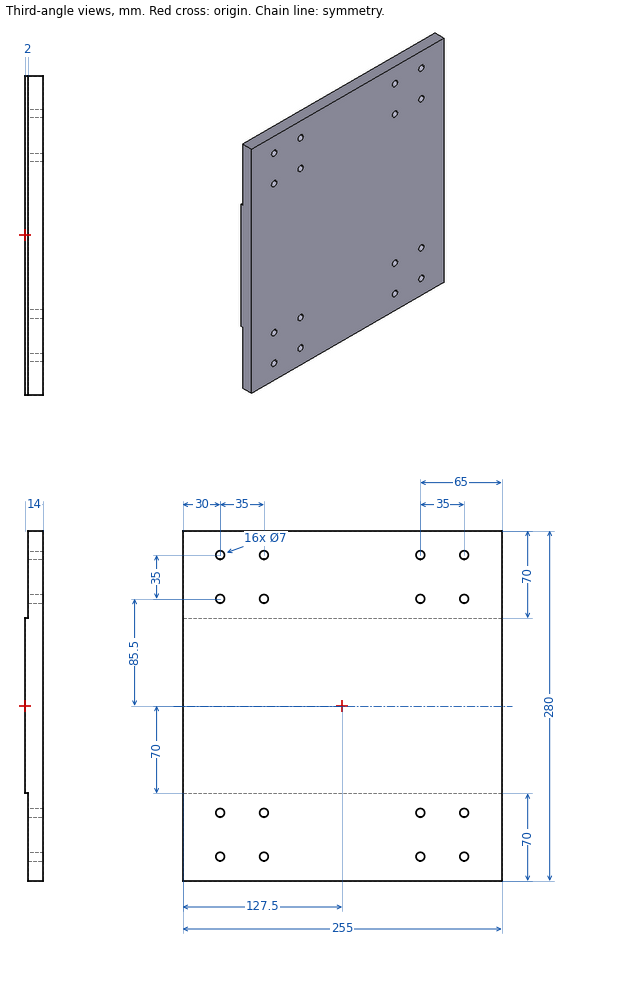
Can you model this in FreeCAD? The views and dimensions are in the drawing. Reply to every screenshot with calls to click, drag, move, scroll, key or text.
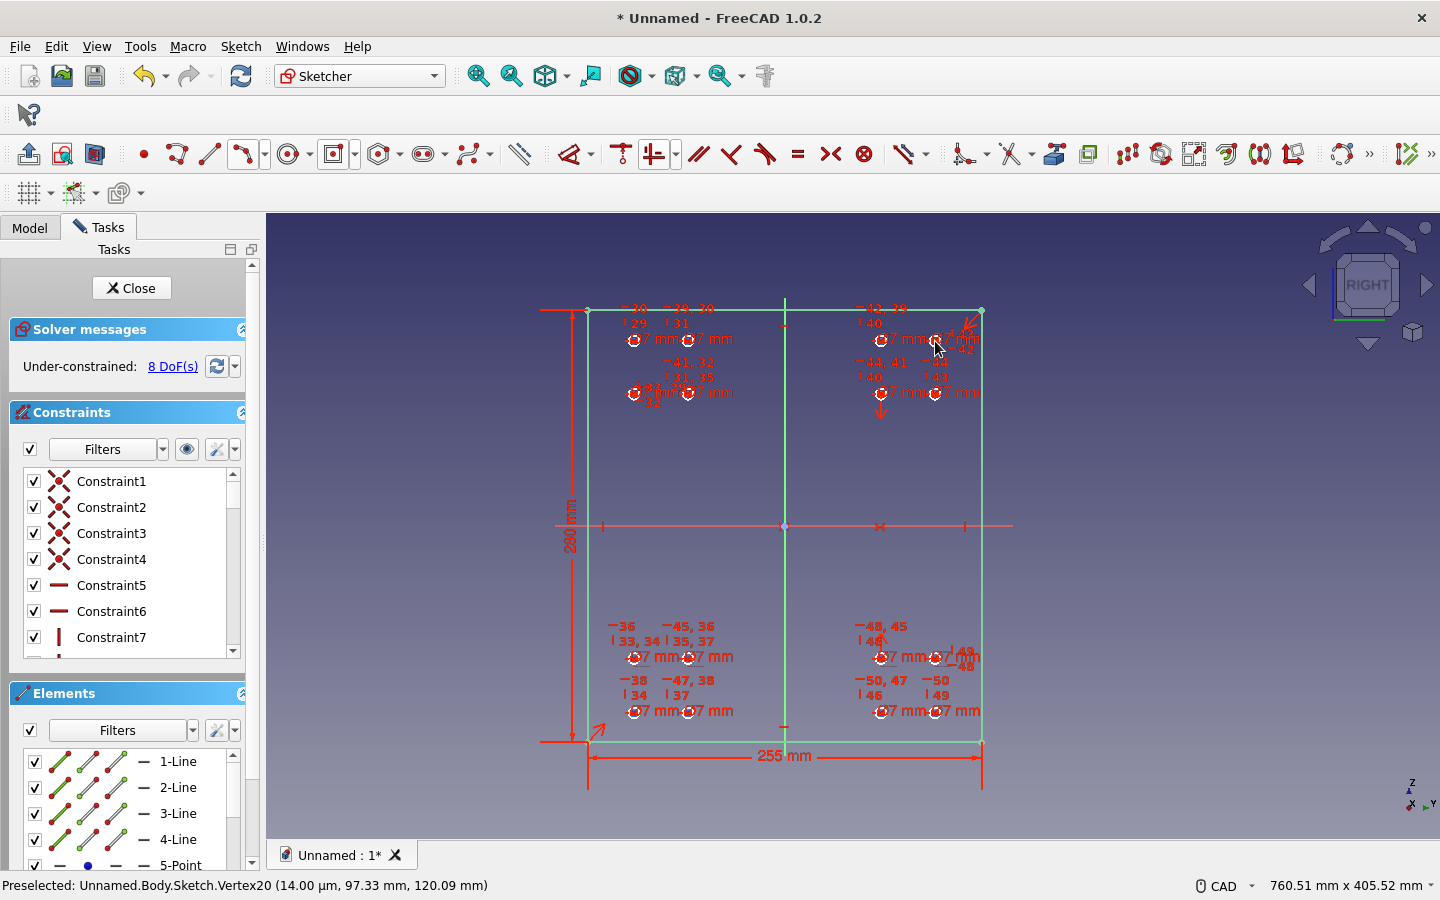
click(935, 713)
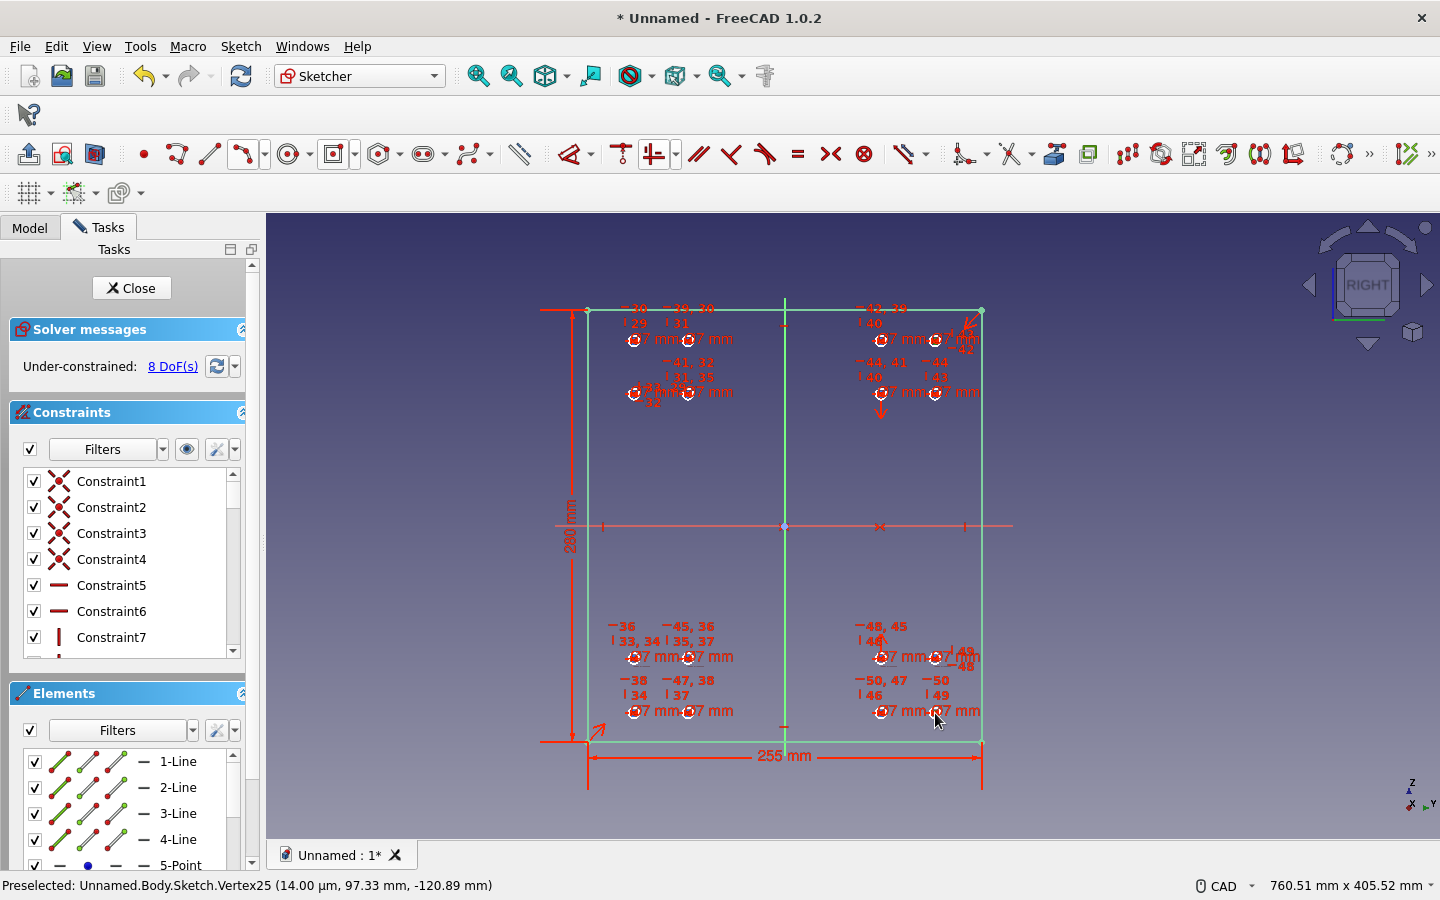
click(644, 526)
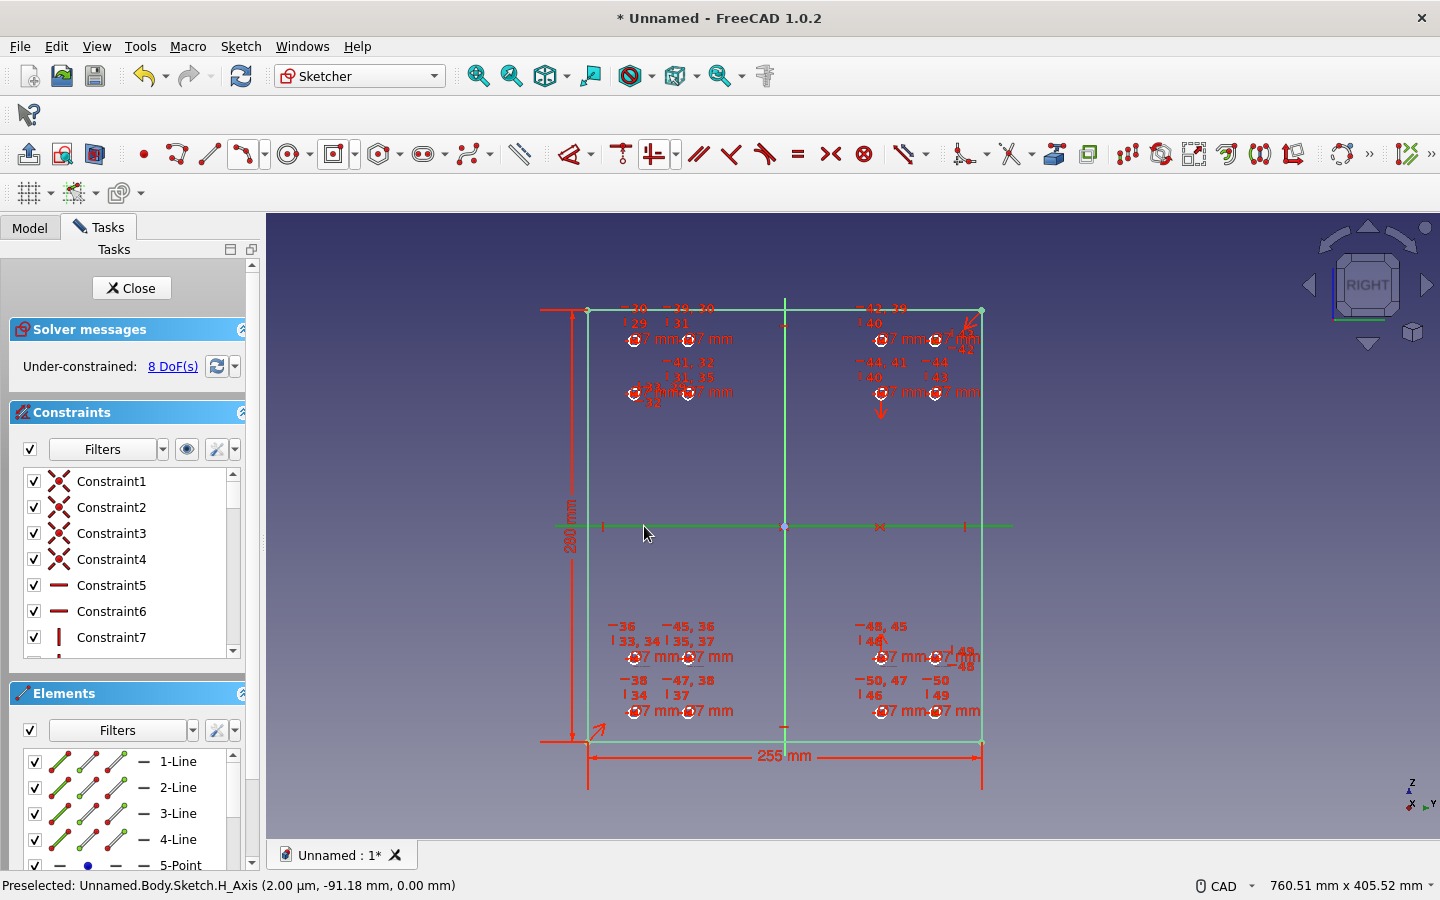
click(831, 154)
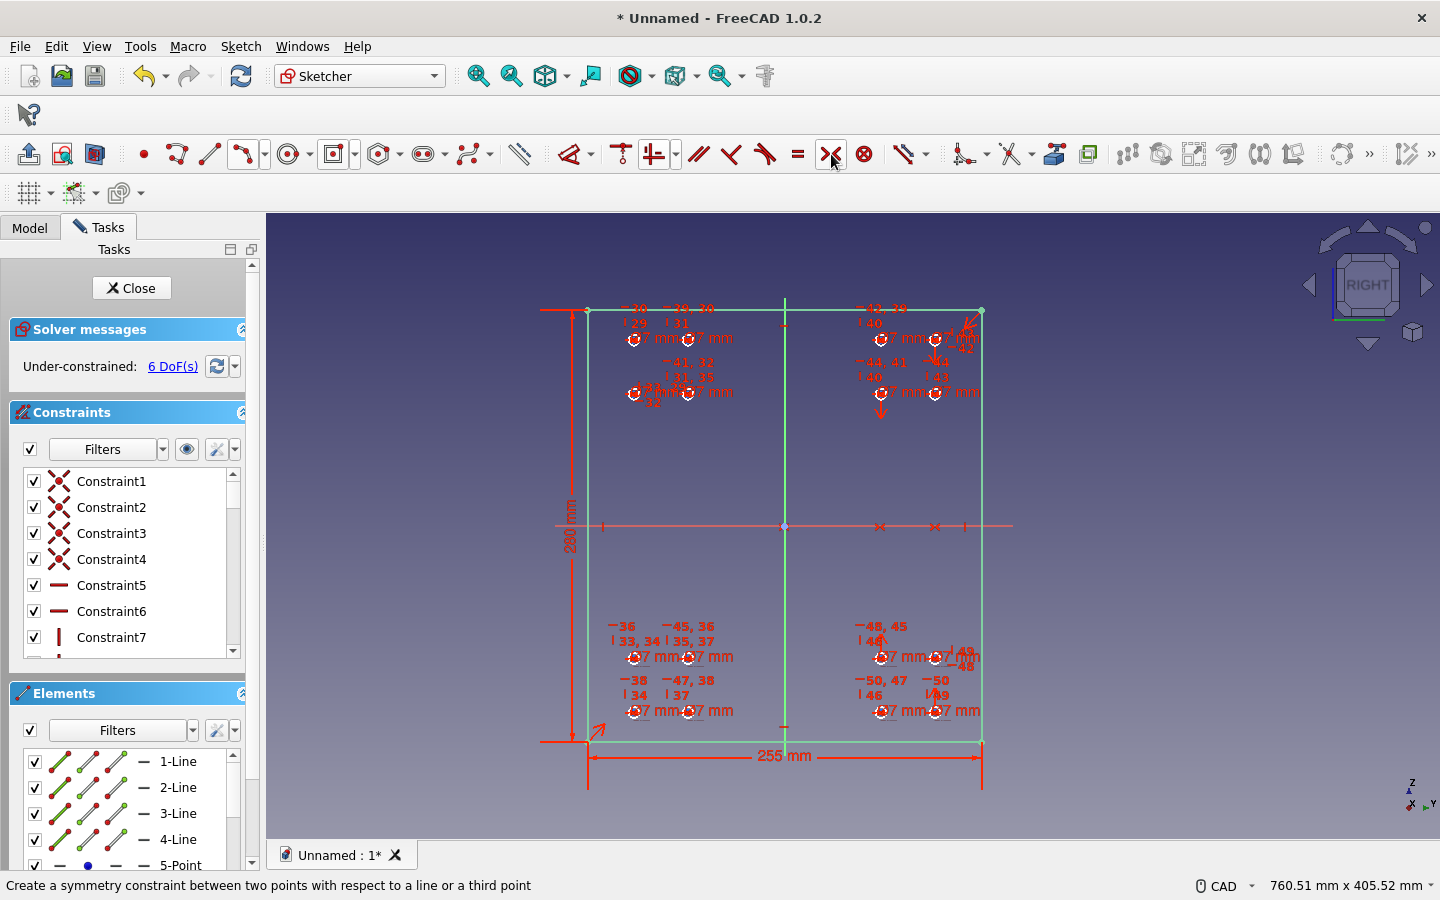
click(588, 310)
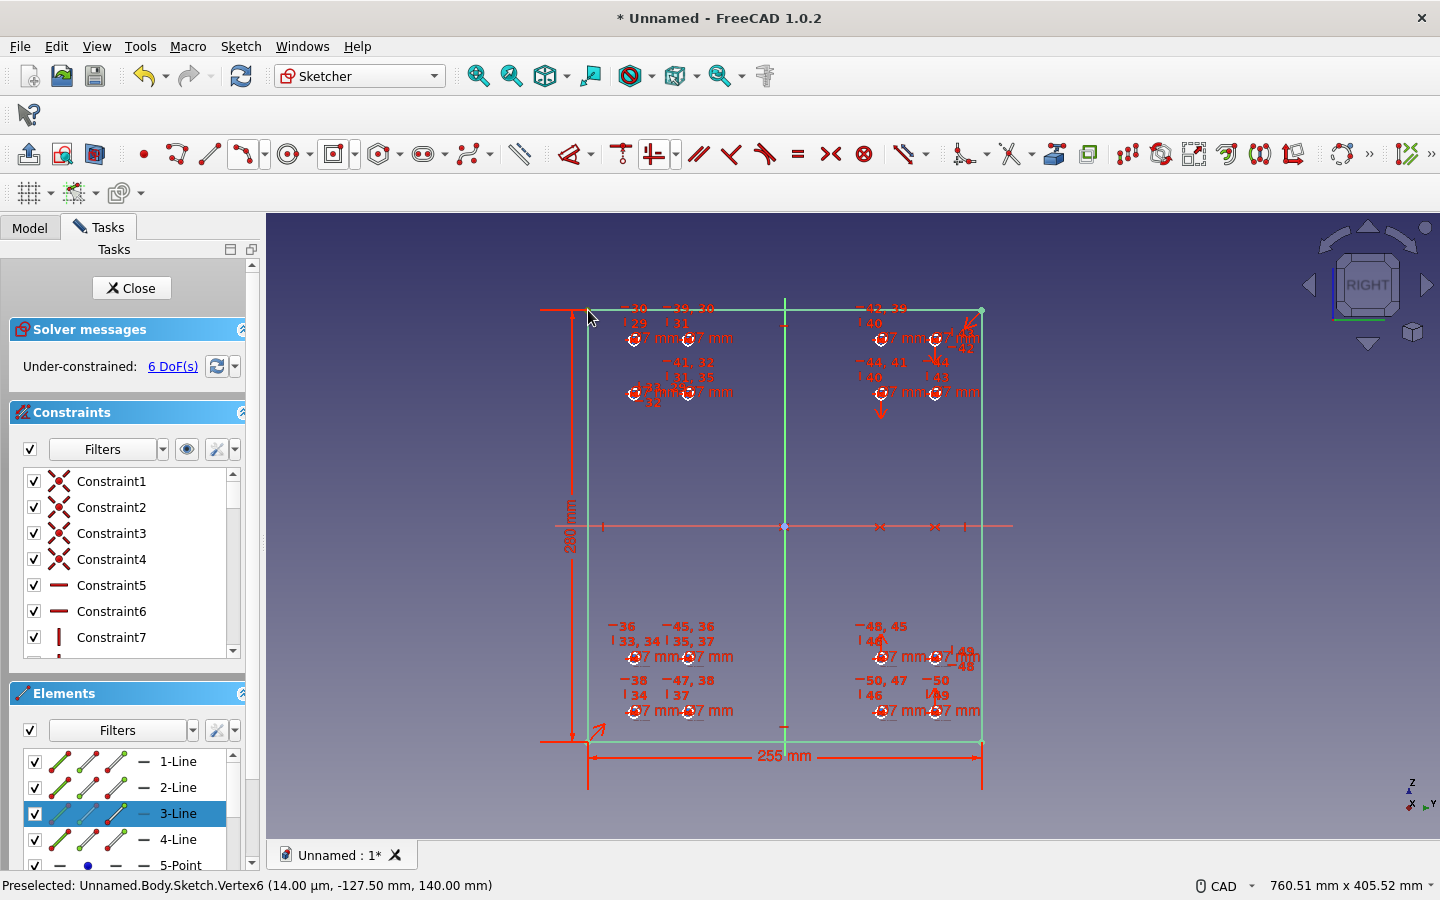
click(634, 340)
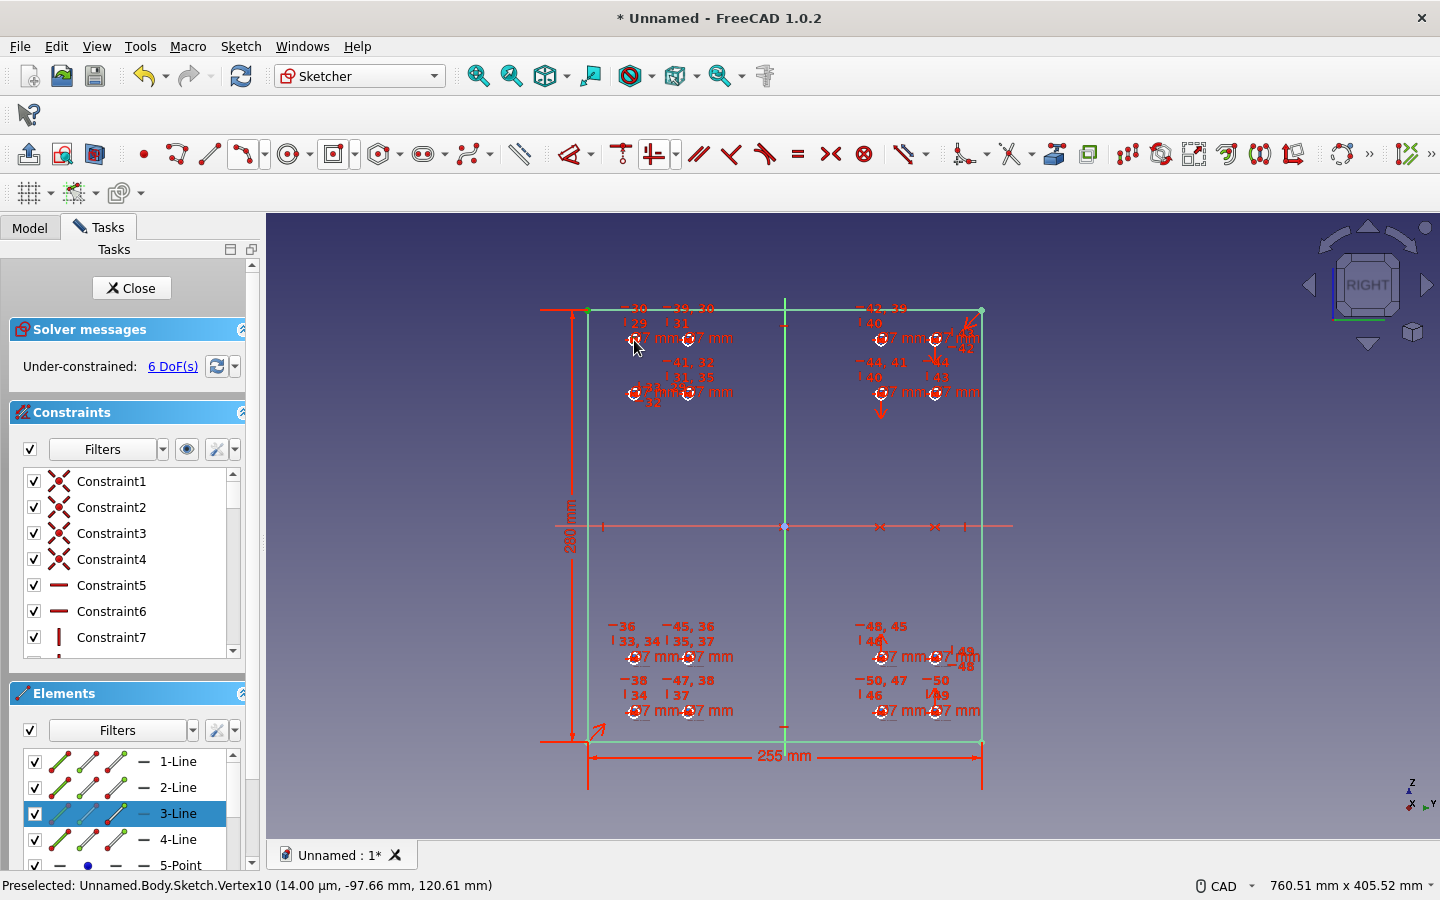
click(590, 154)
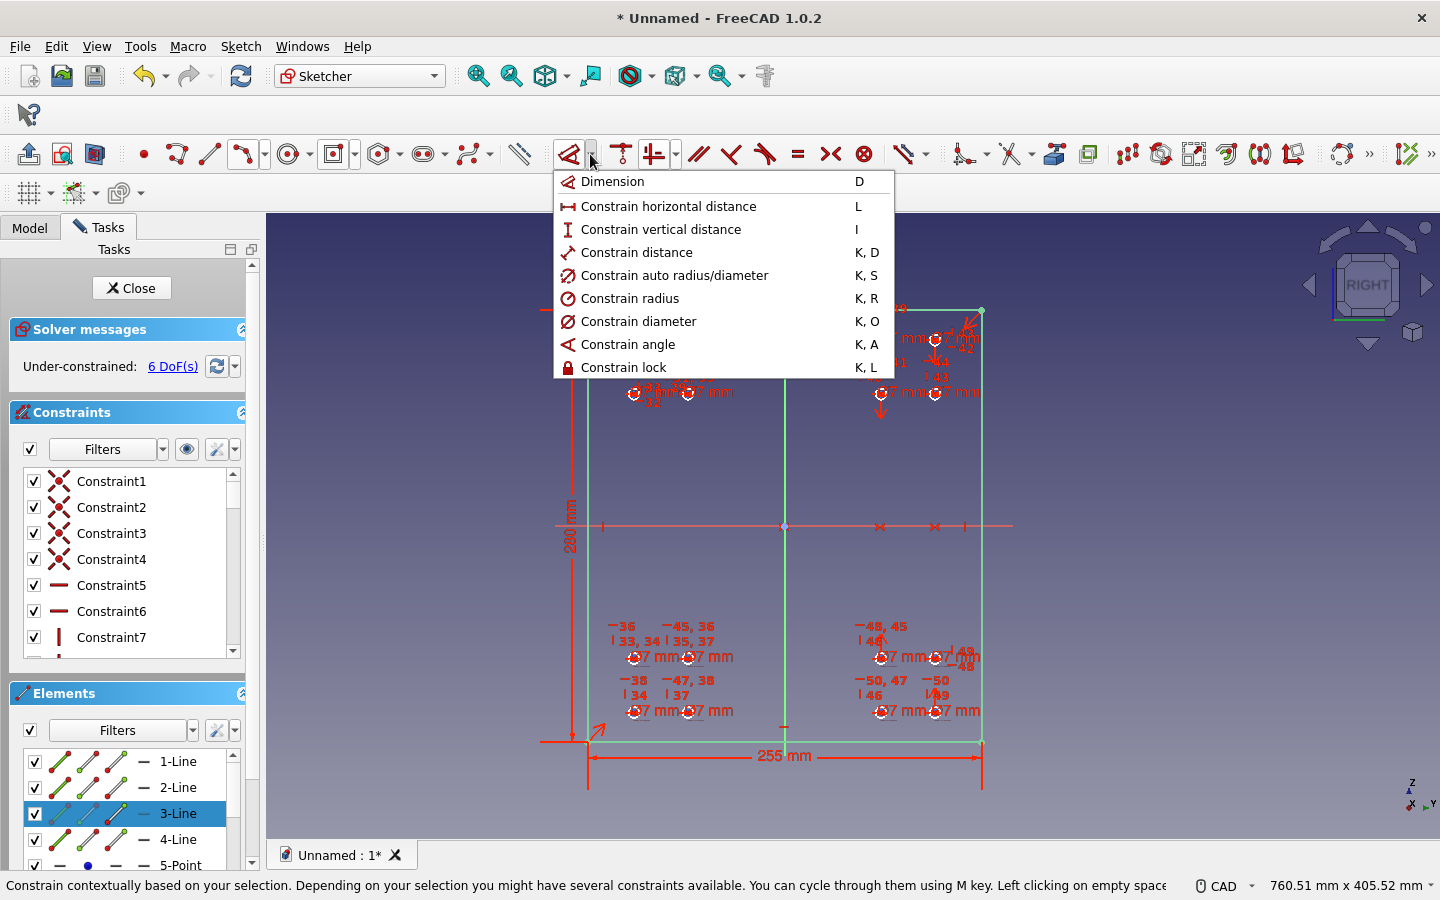
click(724, 206)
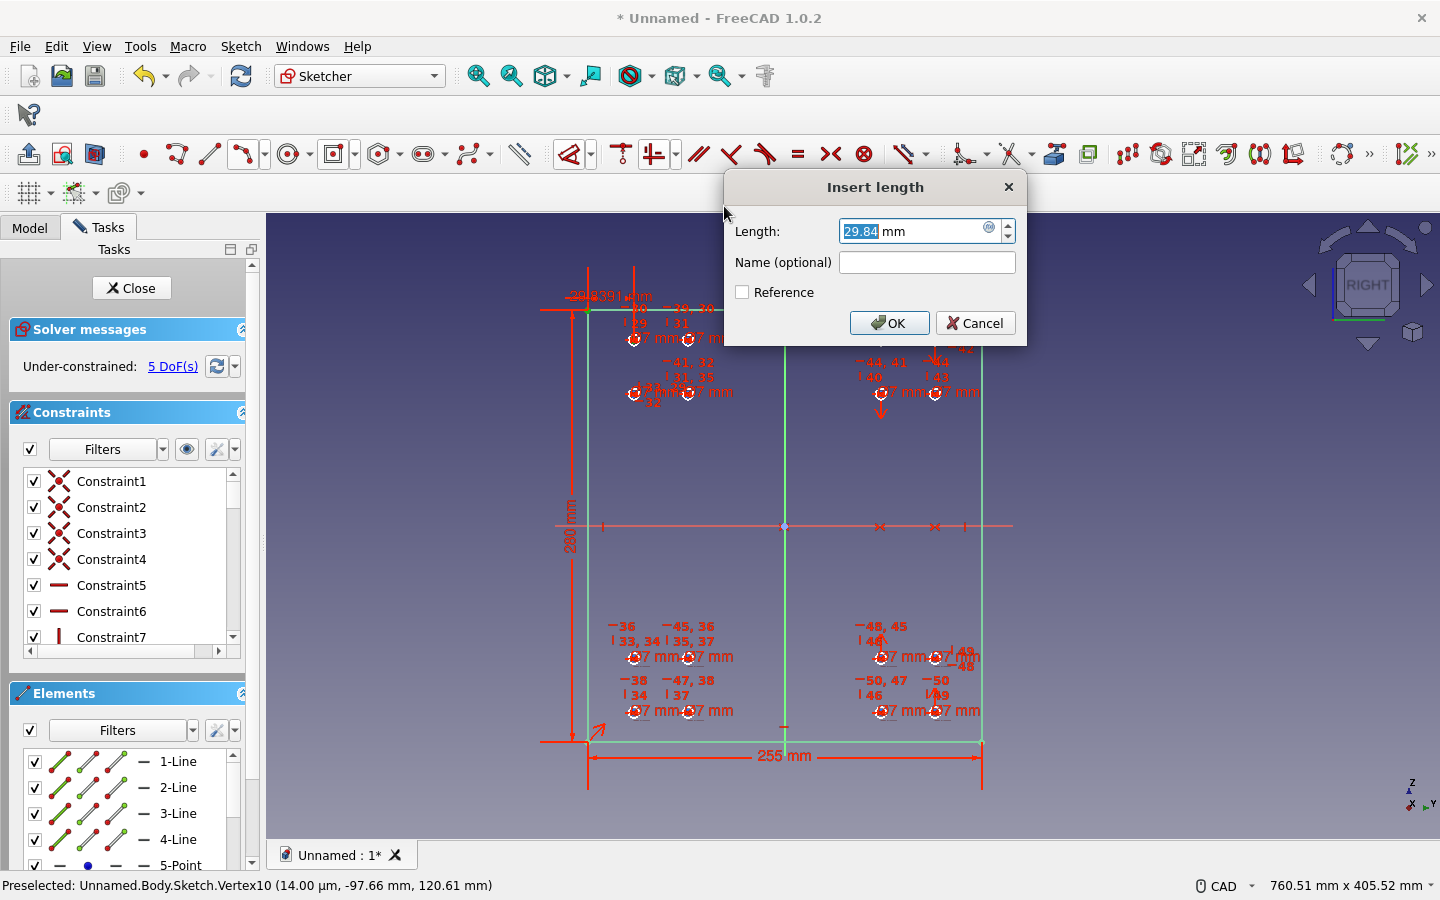
text(30)
key(Return)